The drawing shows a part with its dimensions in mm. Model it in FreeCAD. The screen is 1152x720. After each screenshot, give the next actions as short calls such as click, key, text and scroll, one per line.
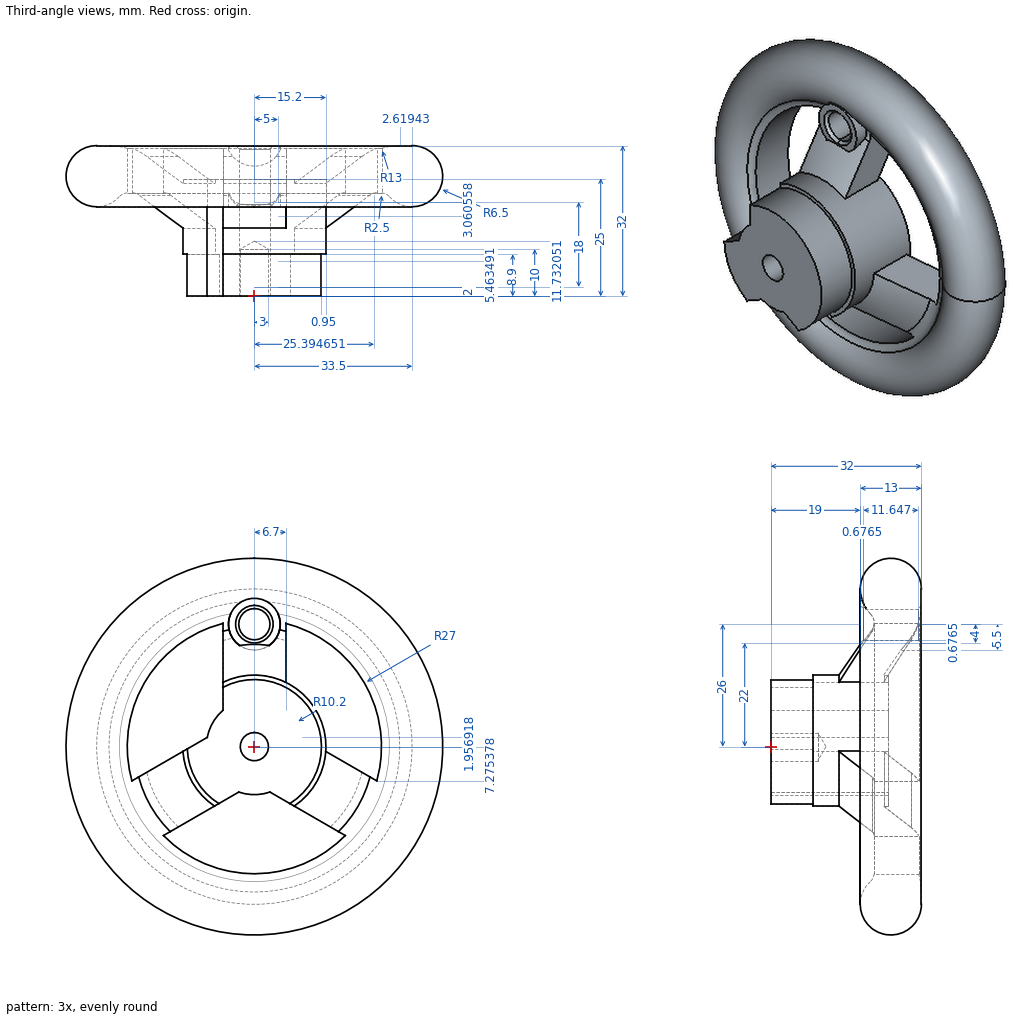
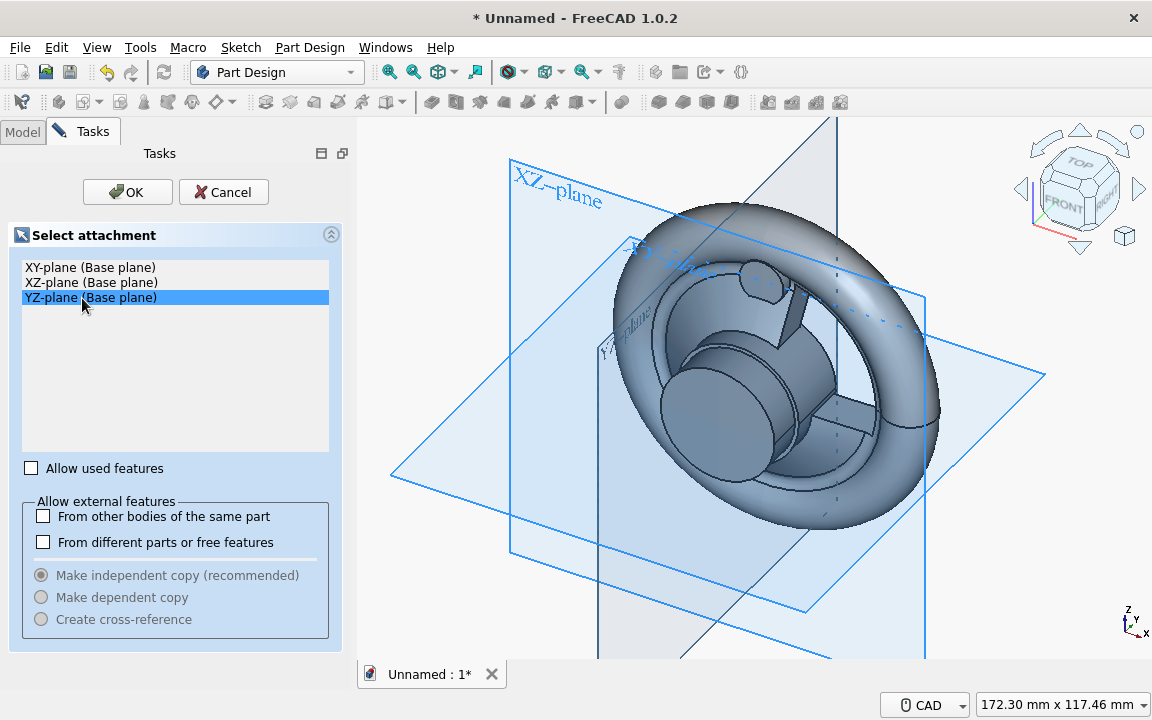
click(128, 192)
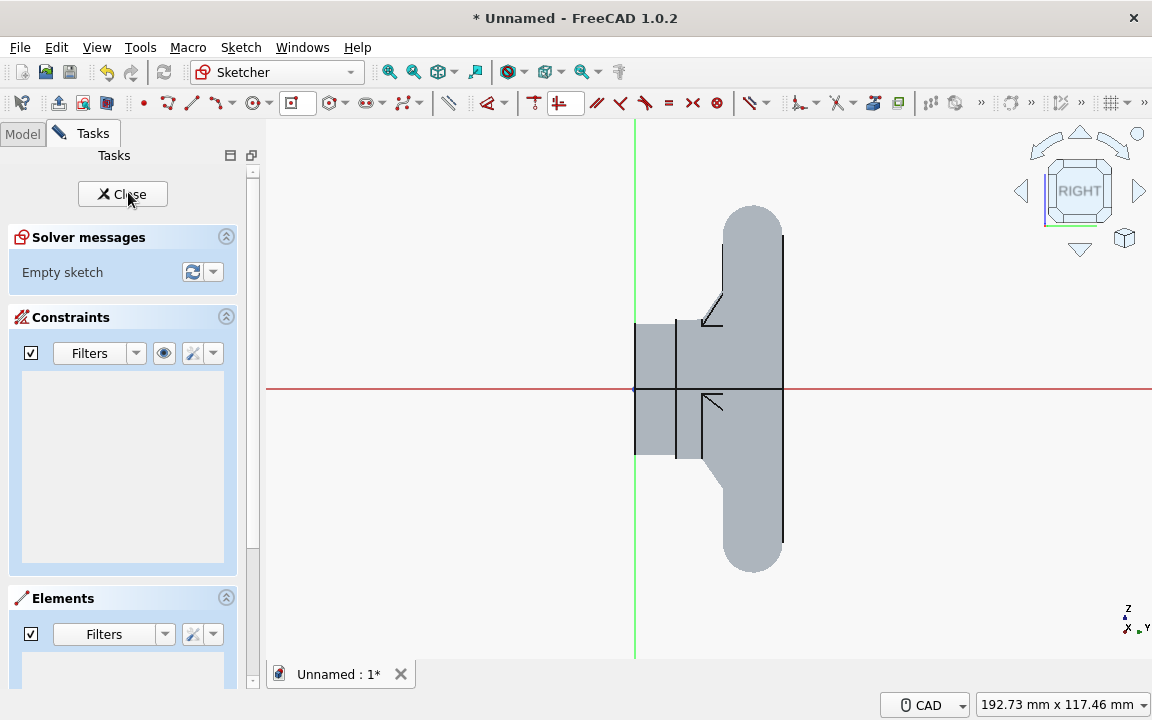
key(q)
key(s)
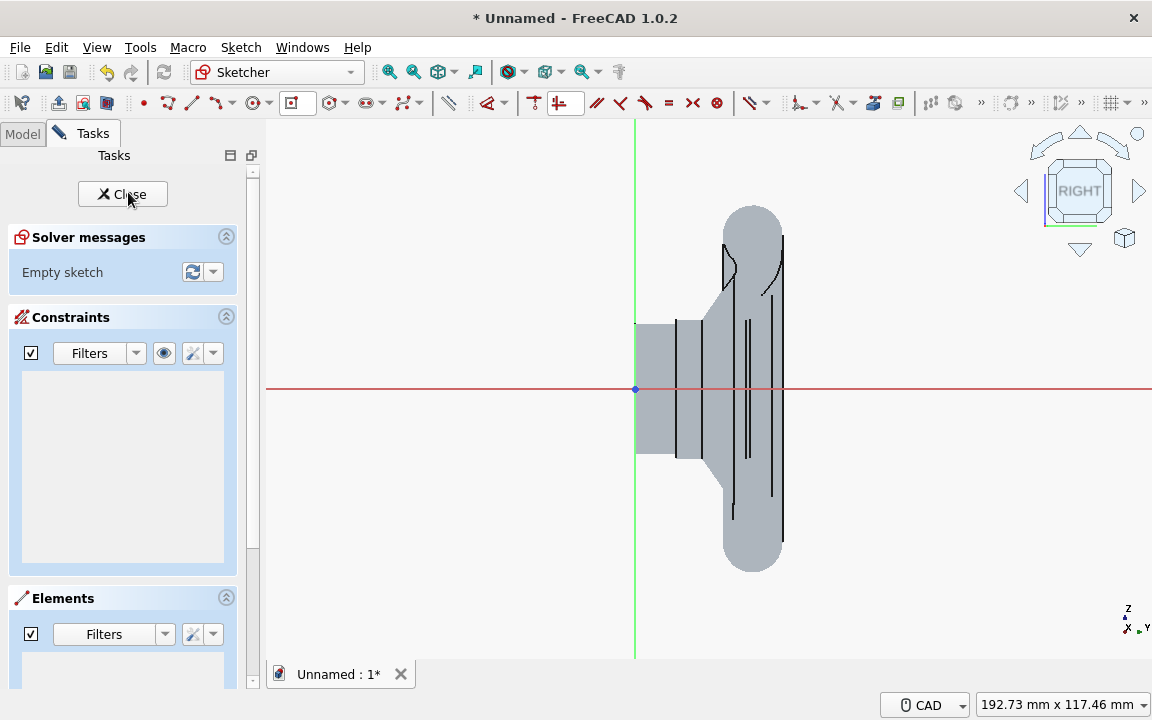
scroll(768, 295, up, 5)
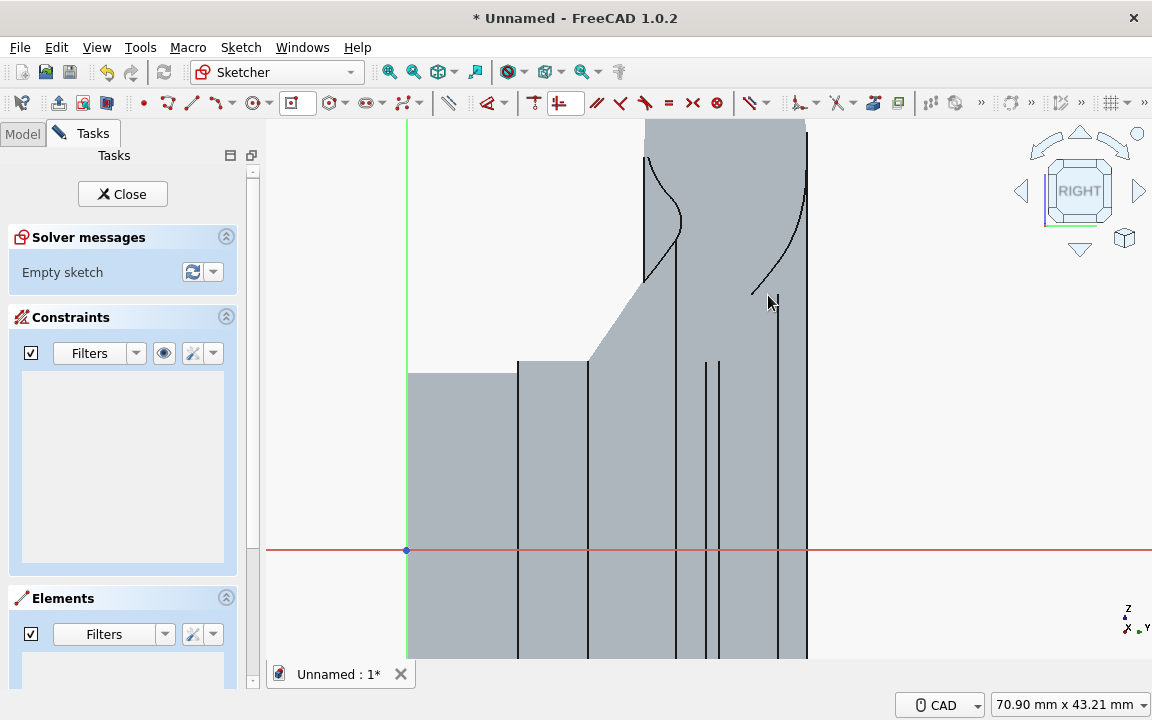
click(168, 104)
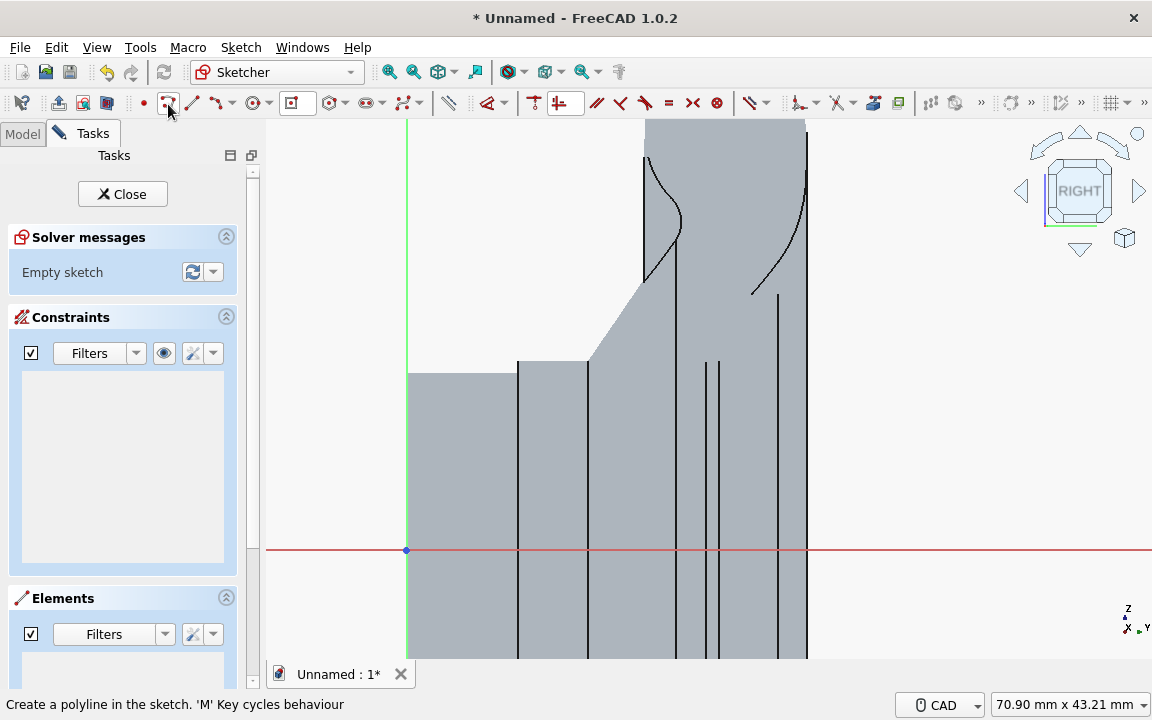
click(644, 275)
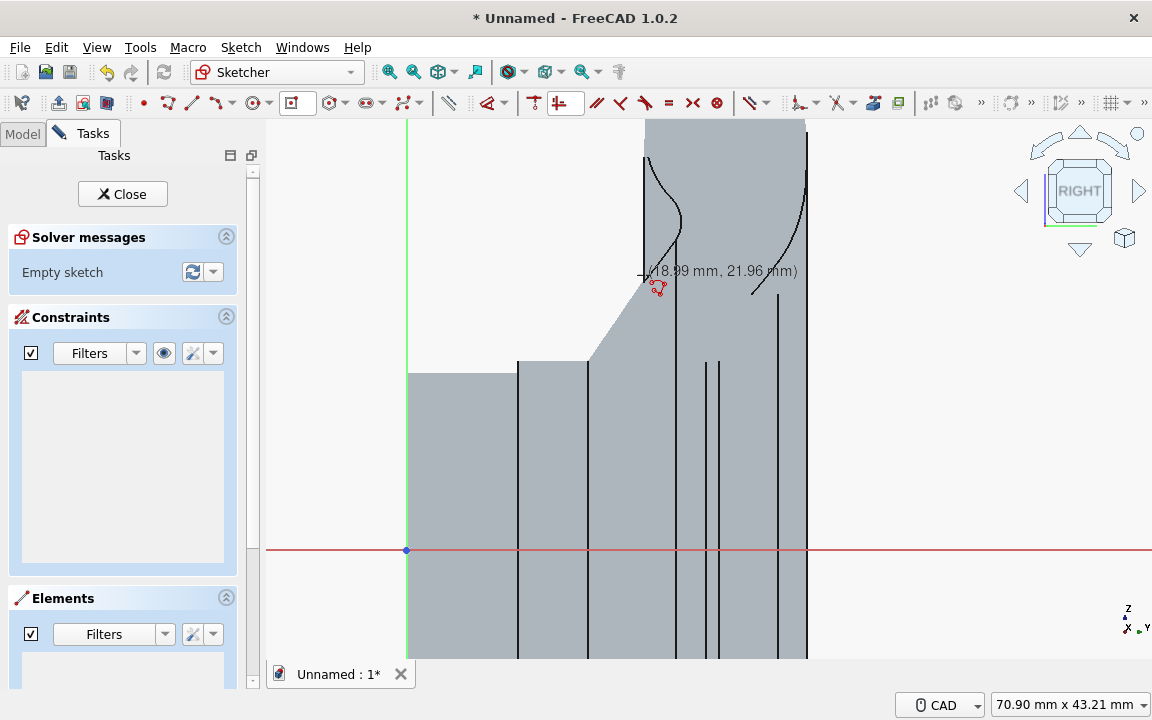
scroll(653, 267, up, 2)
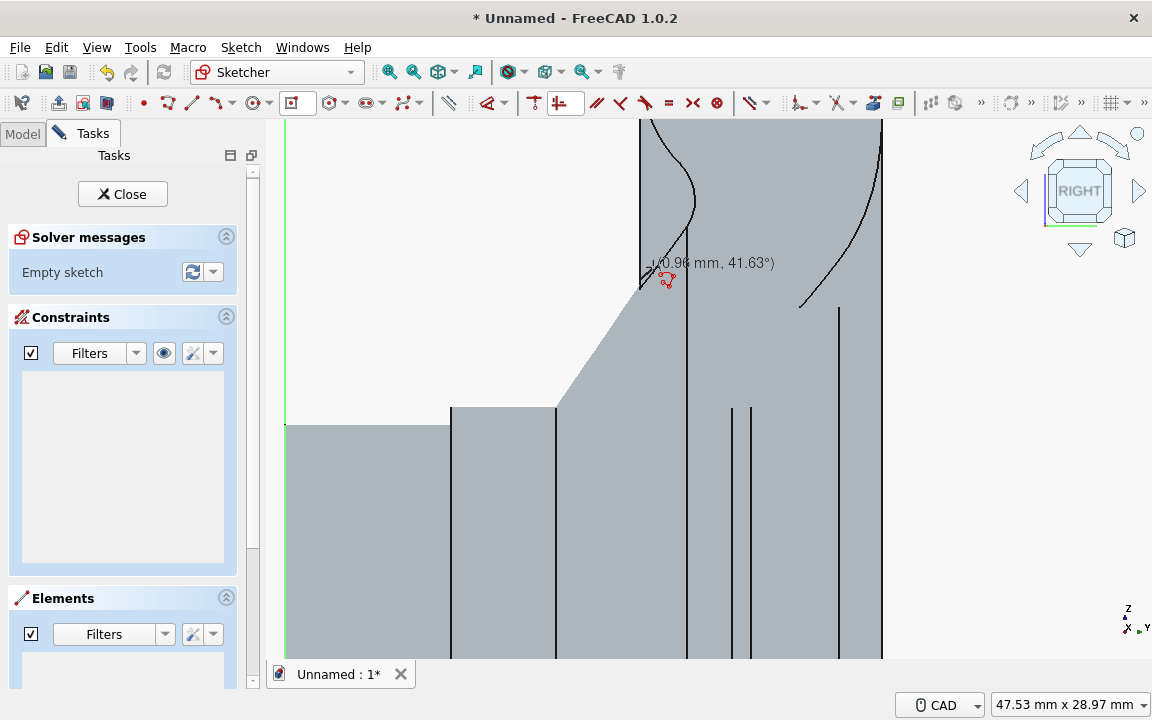
click(652, 267)
click(869, 267)
click(882, 279)
click(882, 205)
click(640, 205)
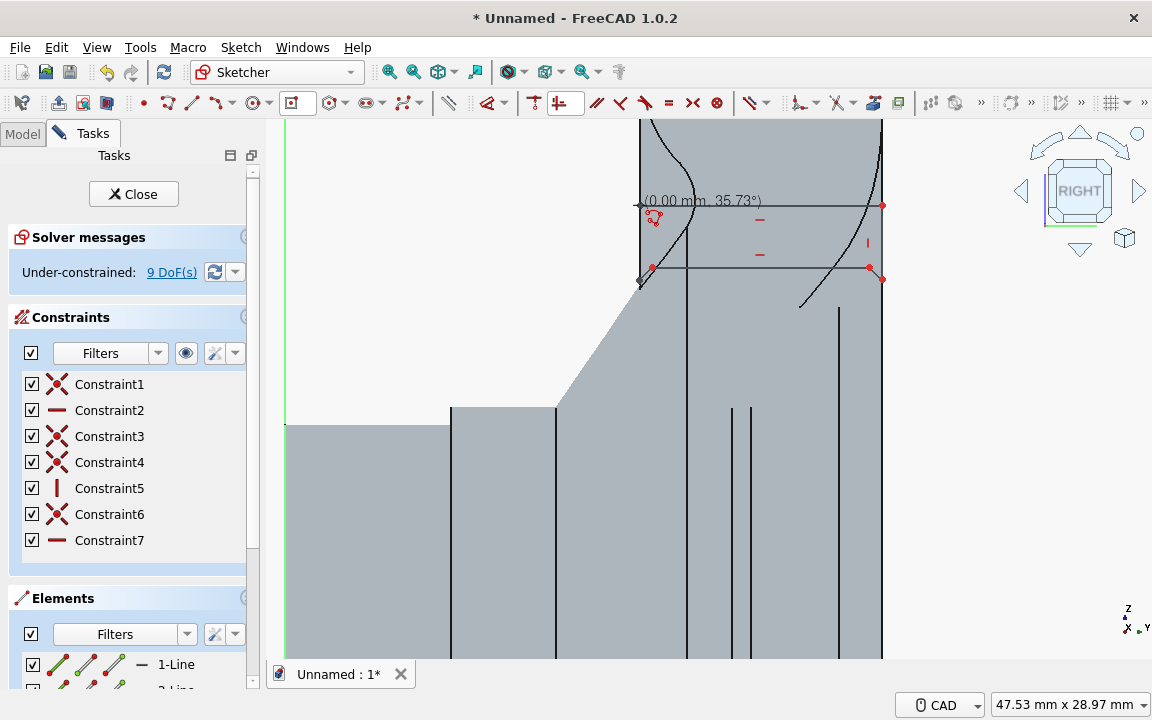
scroll(640, 279, up, 3)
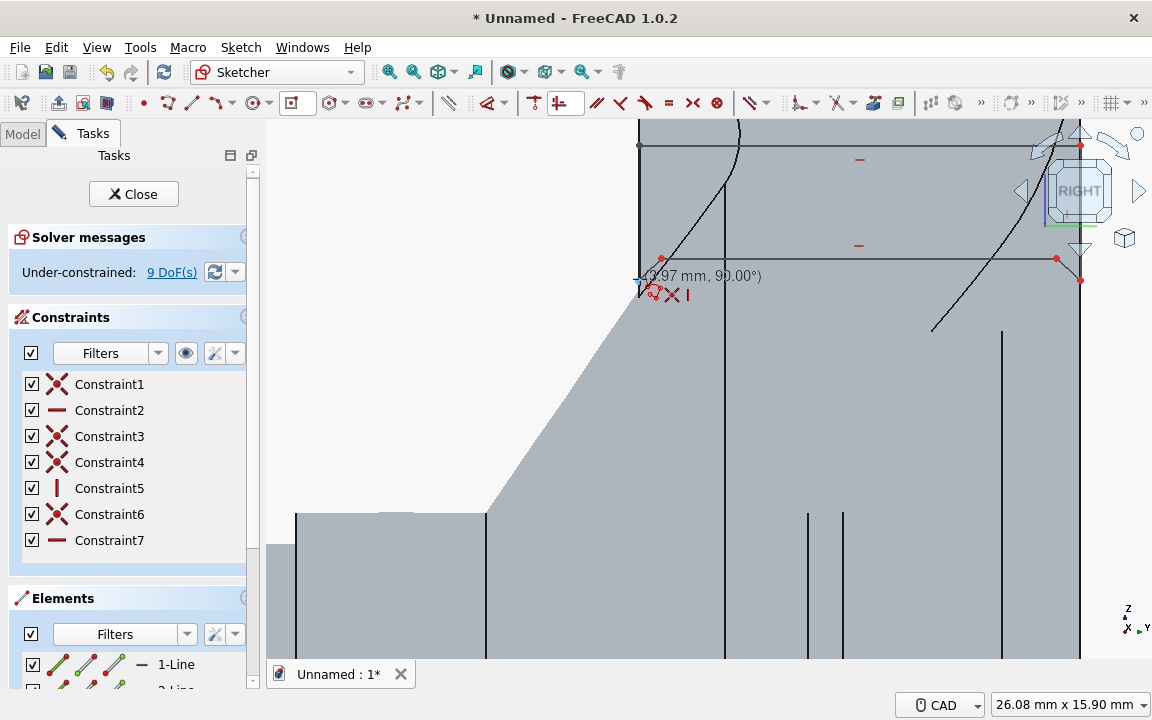
click(638, 281)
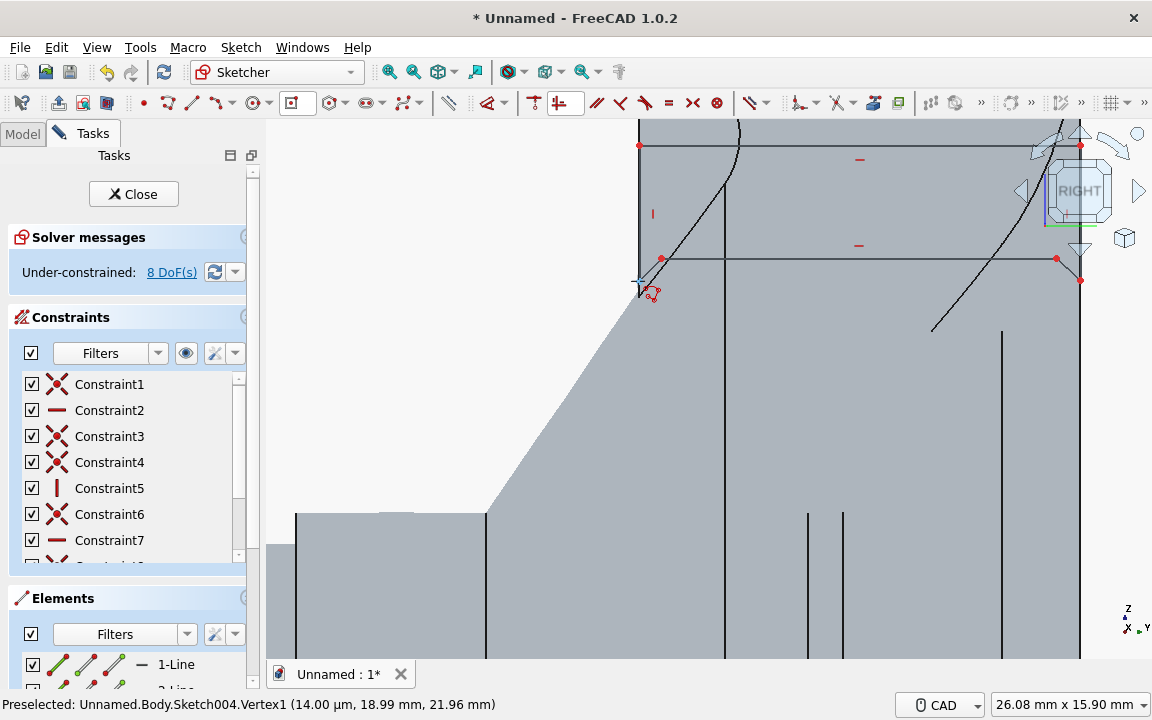
click(192, 104)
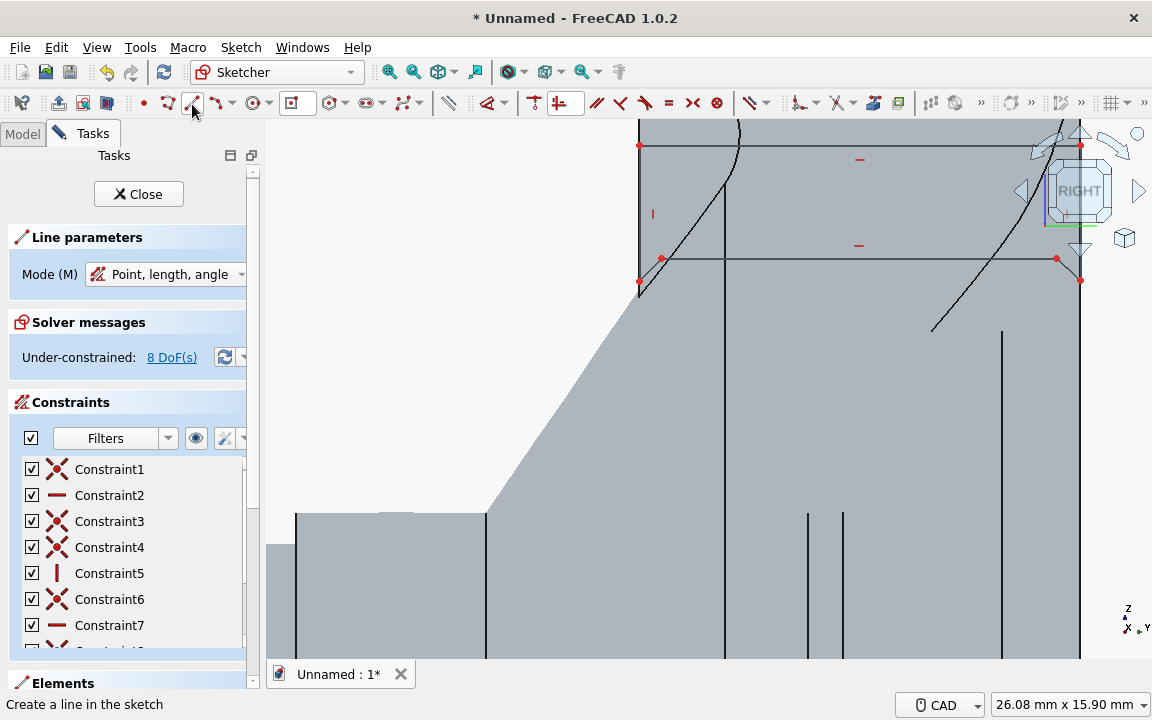
scroll(649, 275, down, 5)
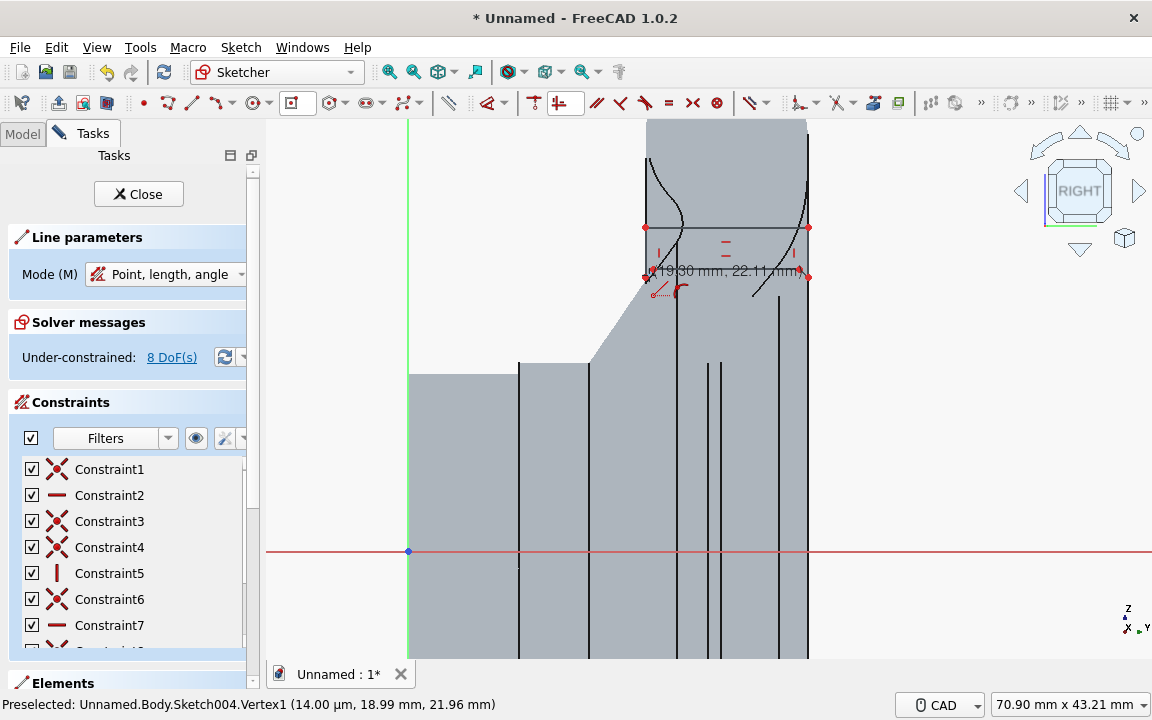
click(824, 227)
click(873, 227)
key(Escape)